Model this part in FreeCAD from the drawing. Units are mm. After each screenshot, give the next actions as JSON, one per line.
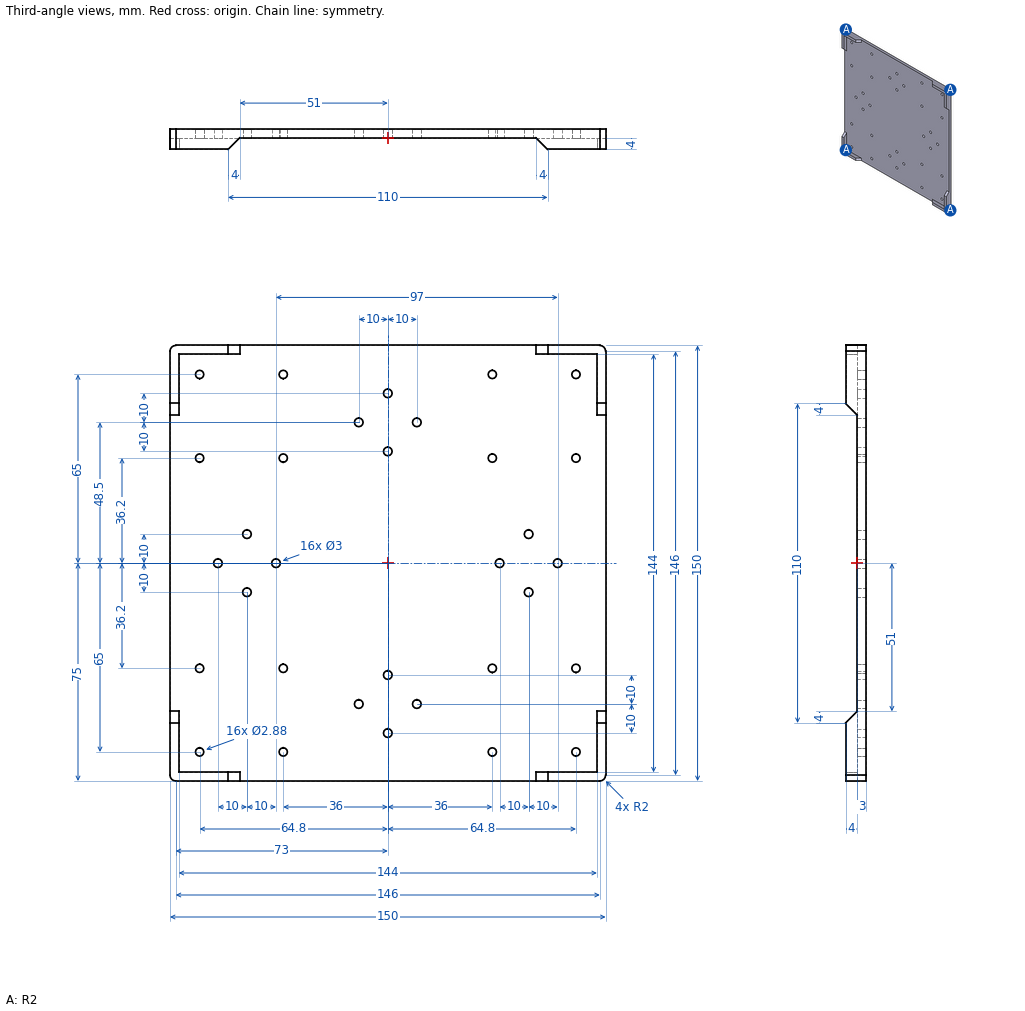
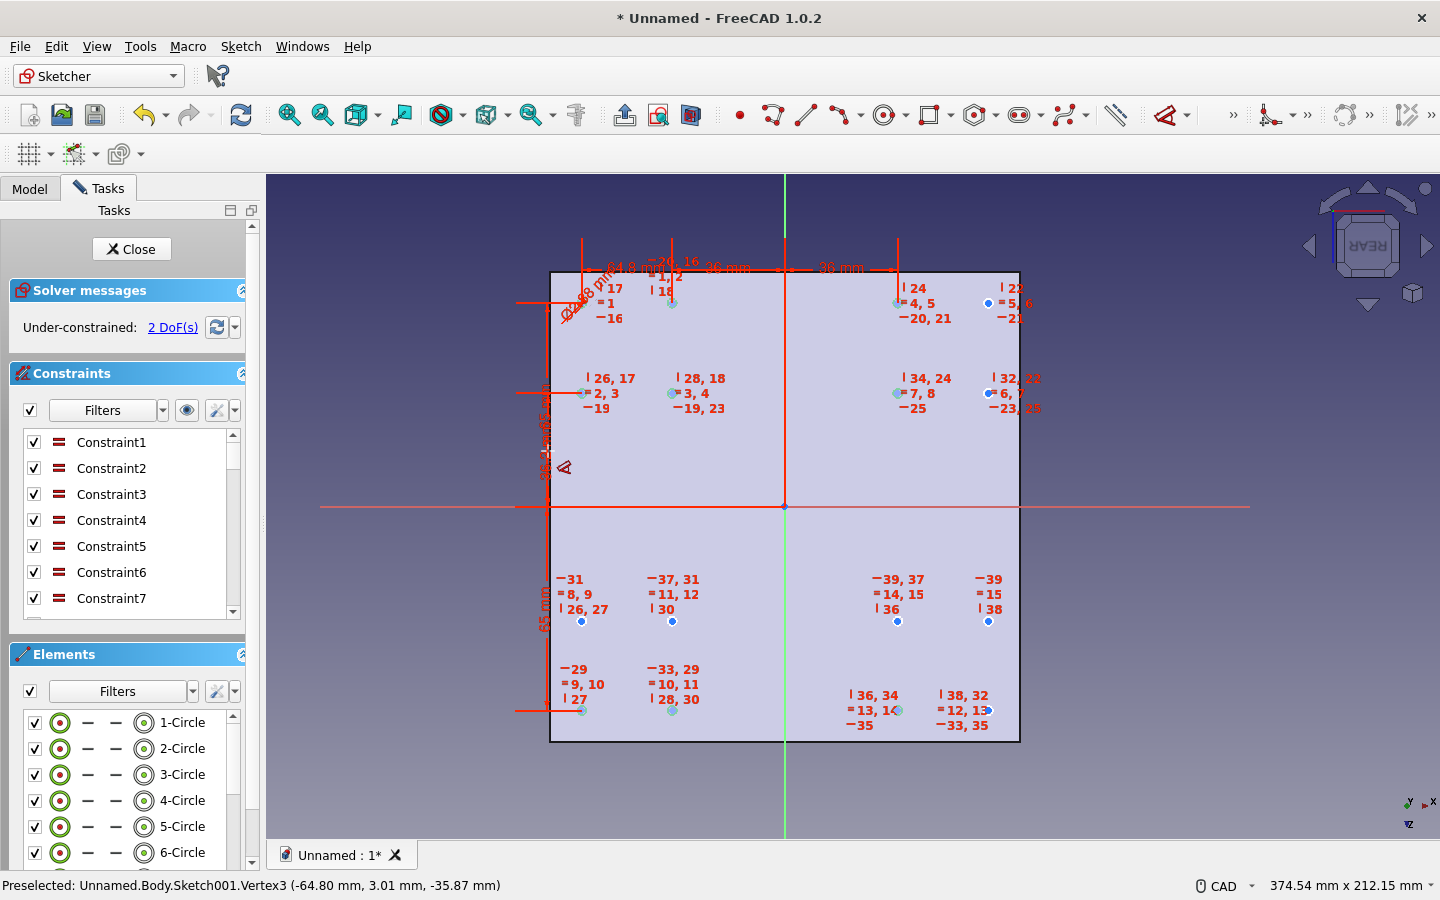
{"action": "left_click", "coordinate": [988, 303]}
{"action": "left_click", "coordinate": [933, 269]}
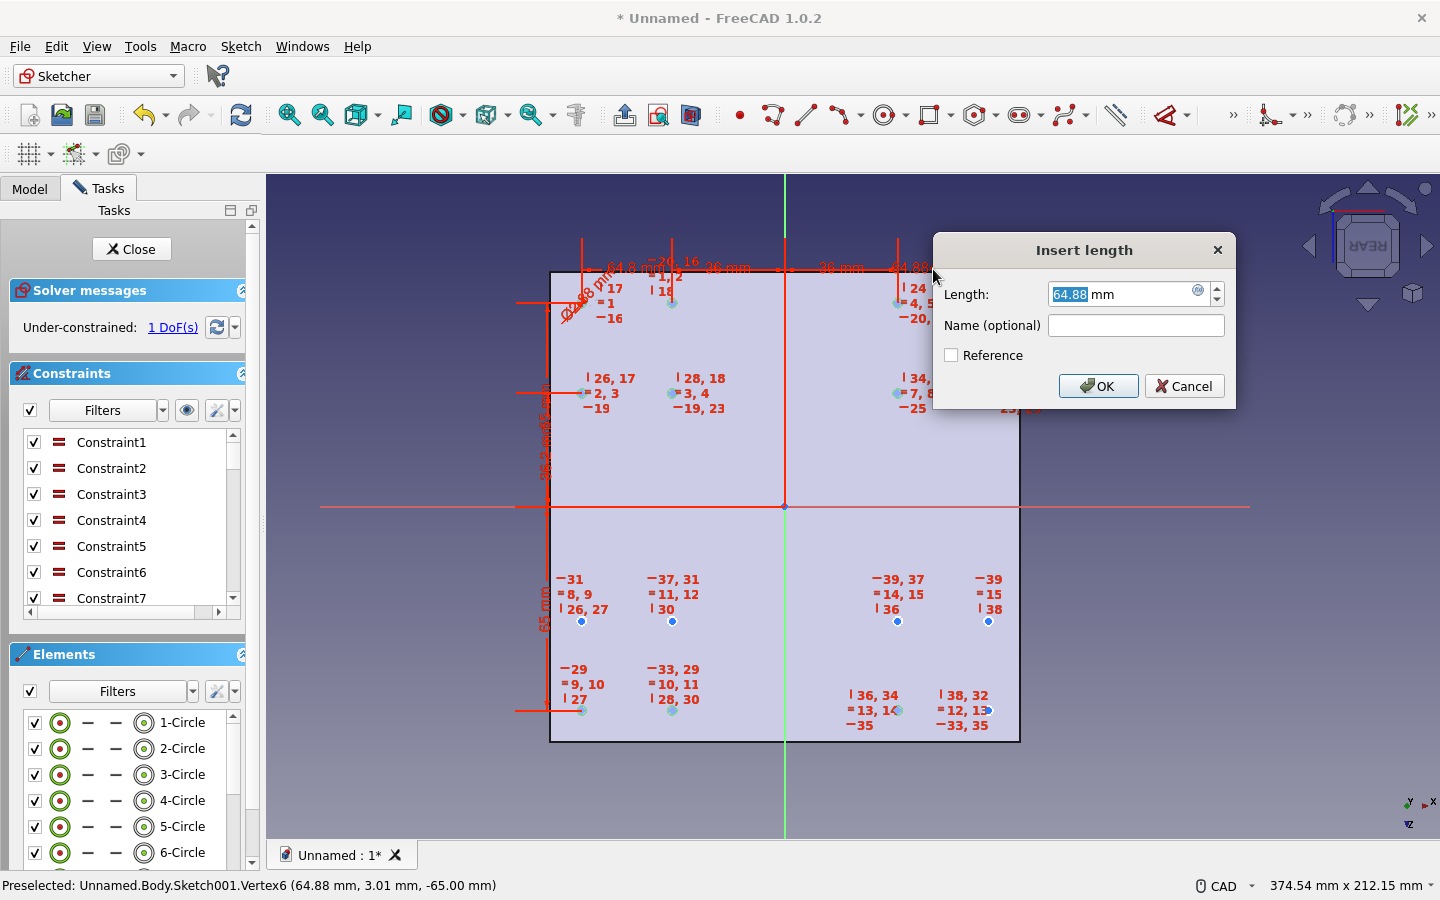
{"action": "type", "text": "64.8"}
{"action": "key", "text": "Return"}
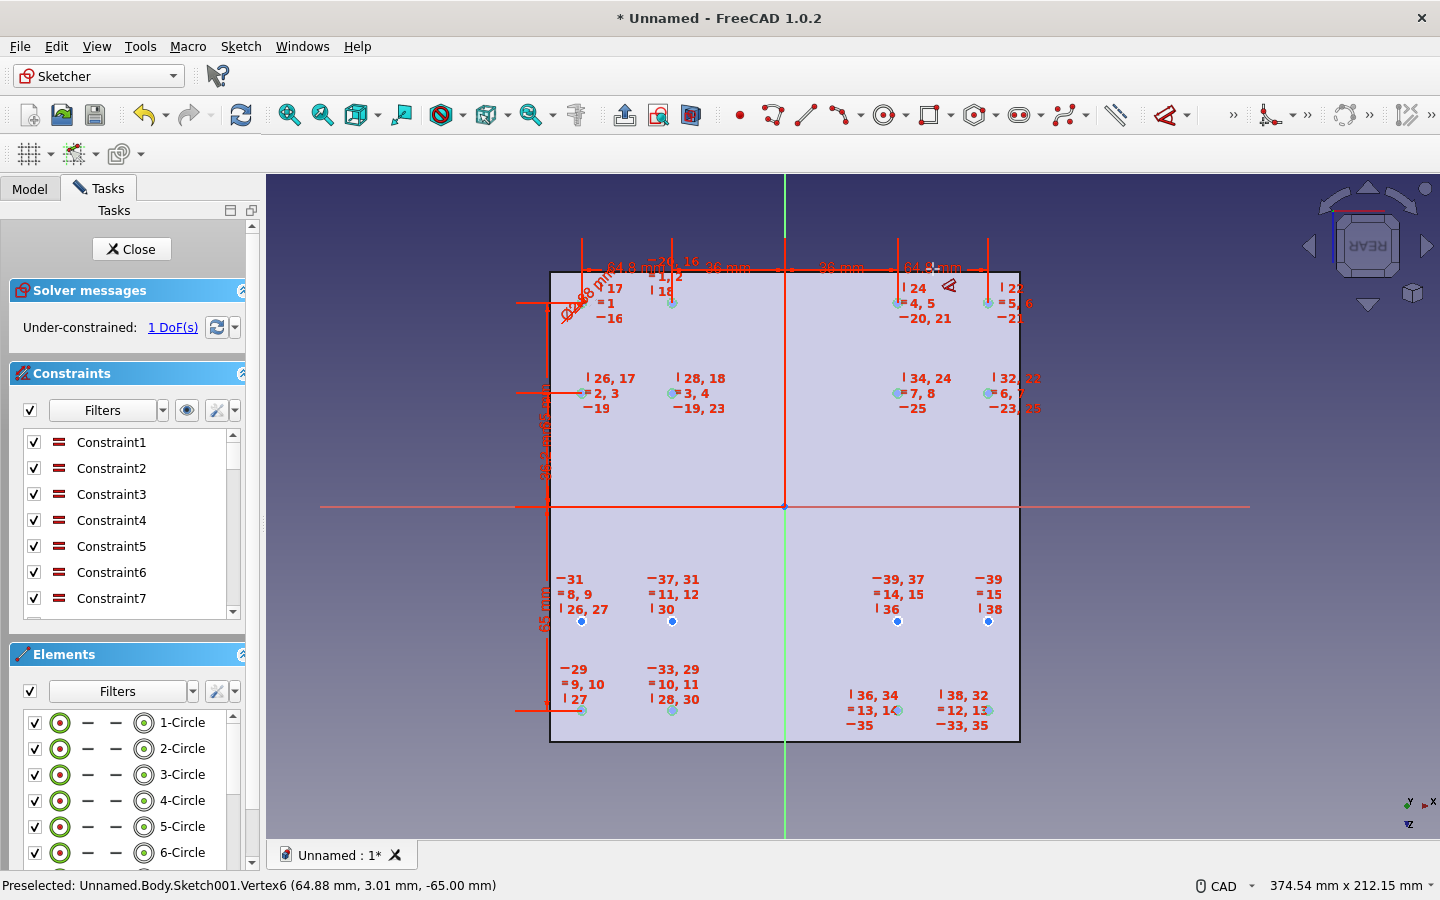
{"action": "left_click", "coordinate": [582, 621]}
{"action": "left_click", "coordinate": [548, 564]}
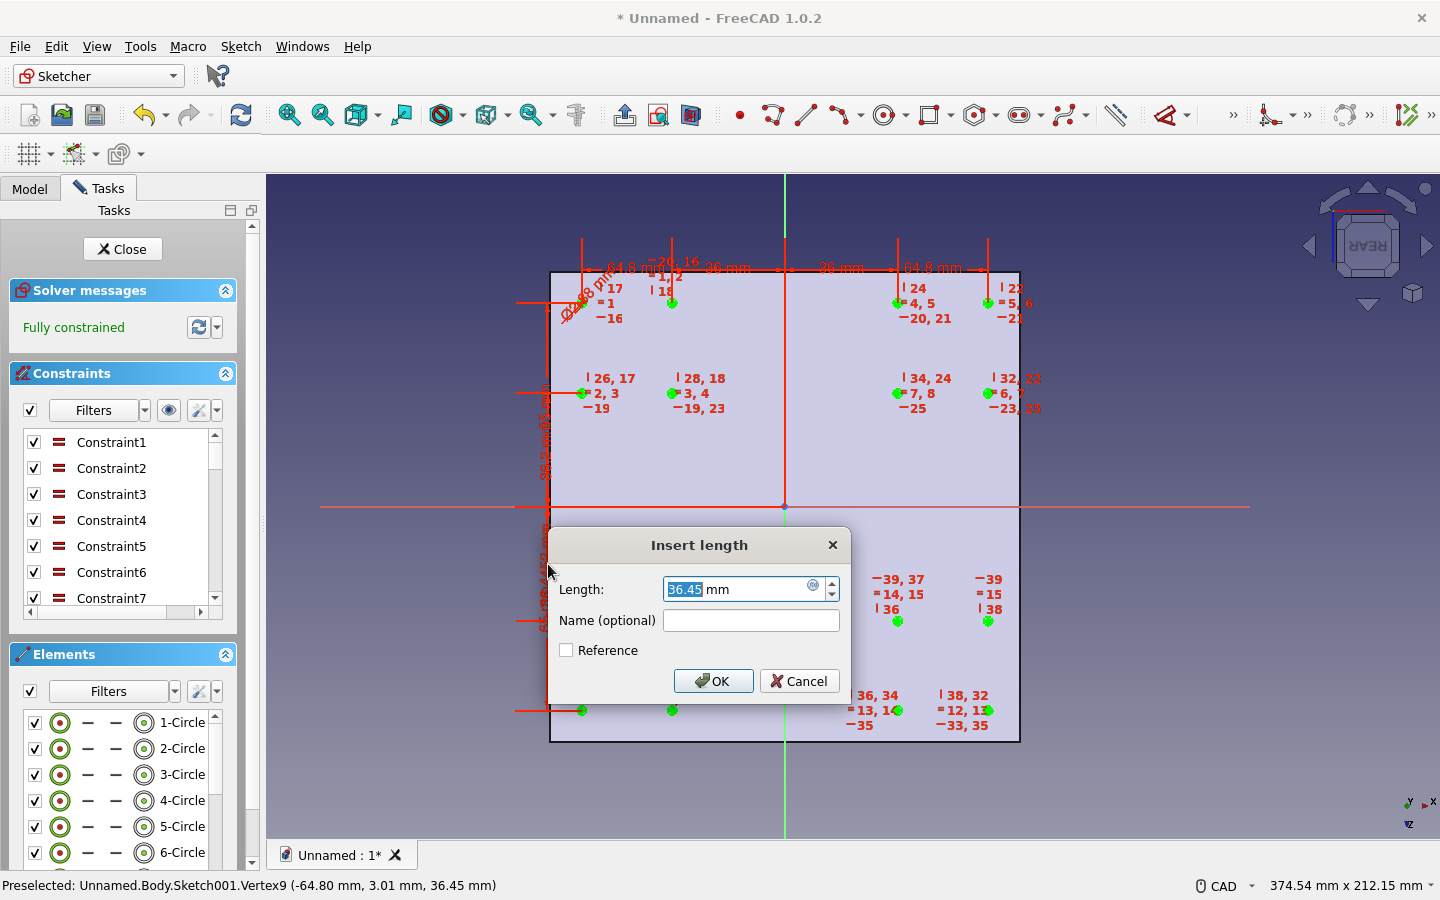
{"action": "type", "text": "36.2"}
{"action": "key", "text": "Return"}
{"action": "key", "text": "Escape"}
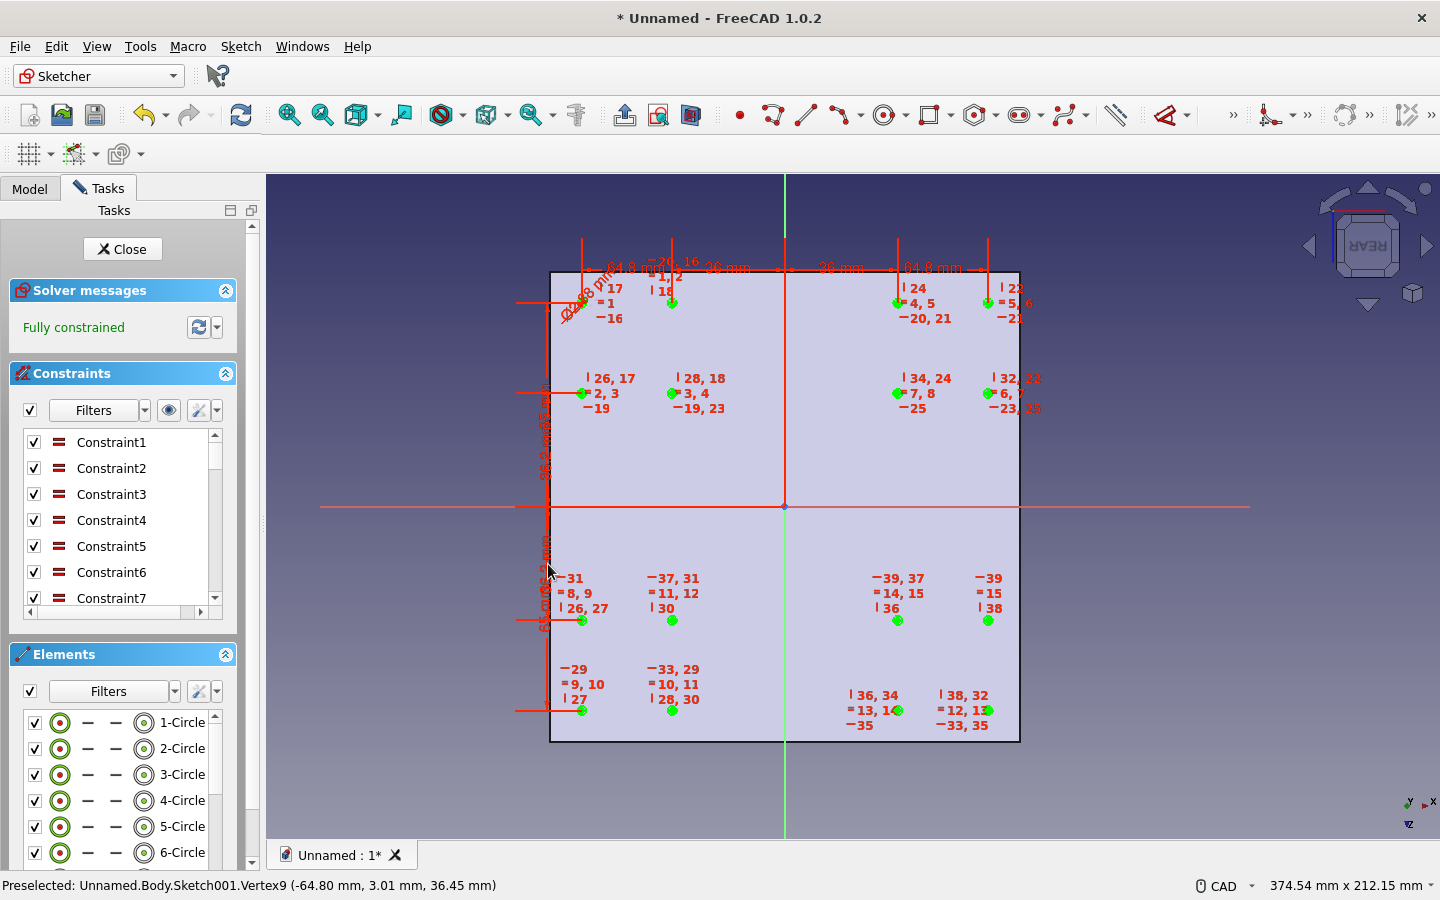
{"action": "left_click", "coordinate": [123, 249]}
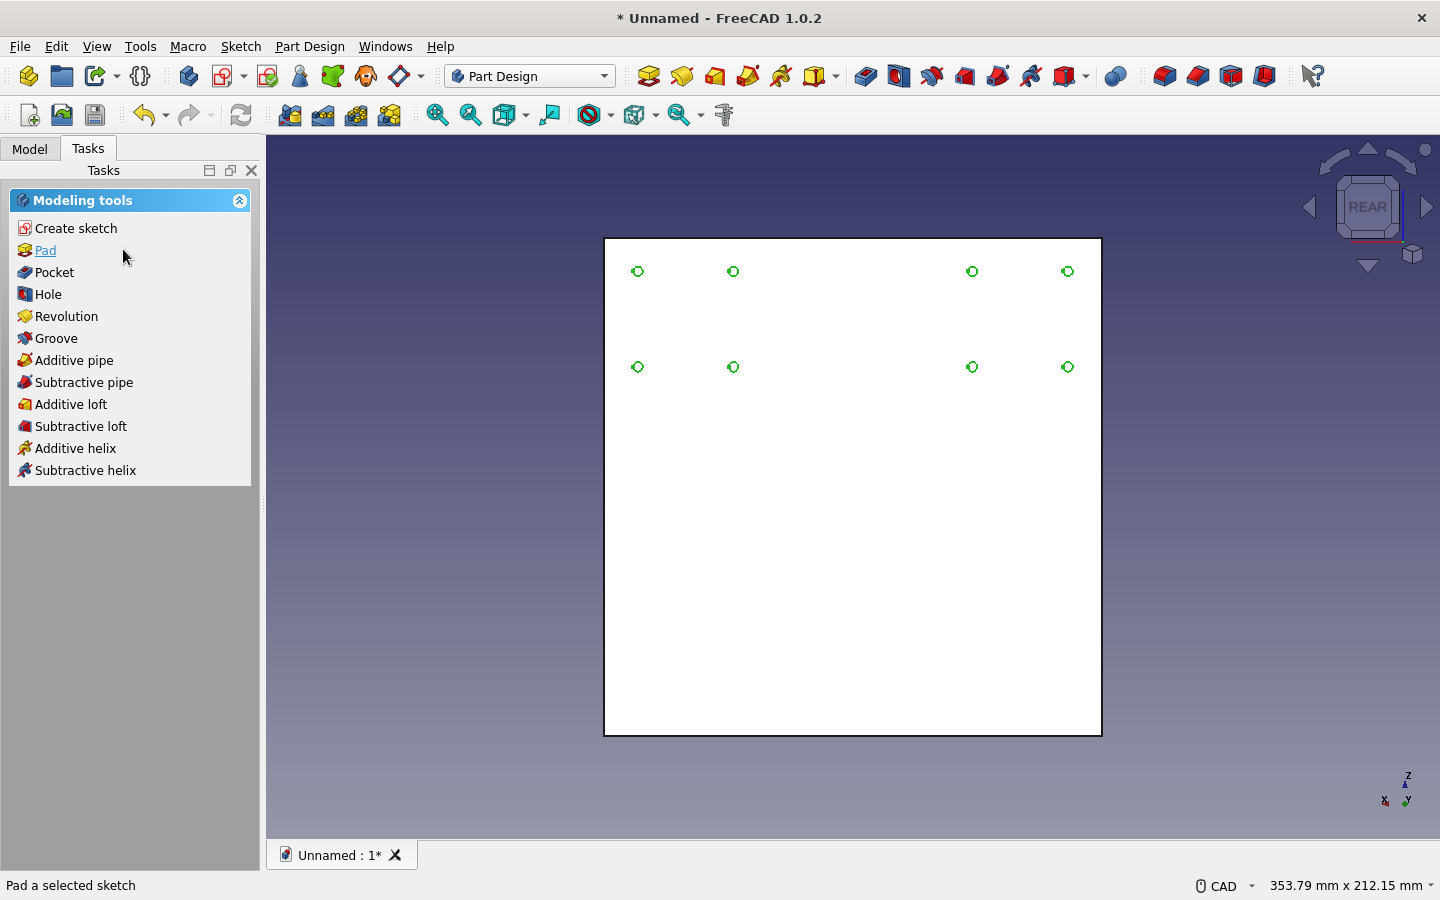
{"action": "left_click", "coordinate": [866, 76]}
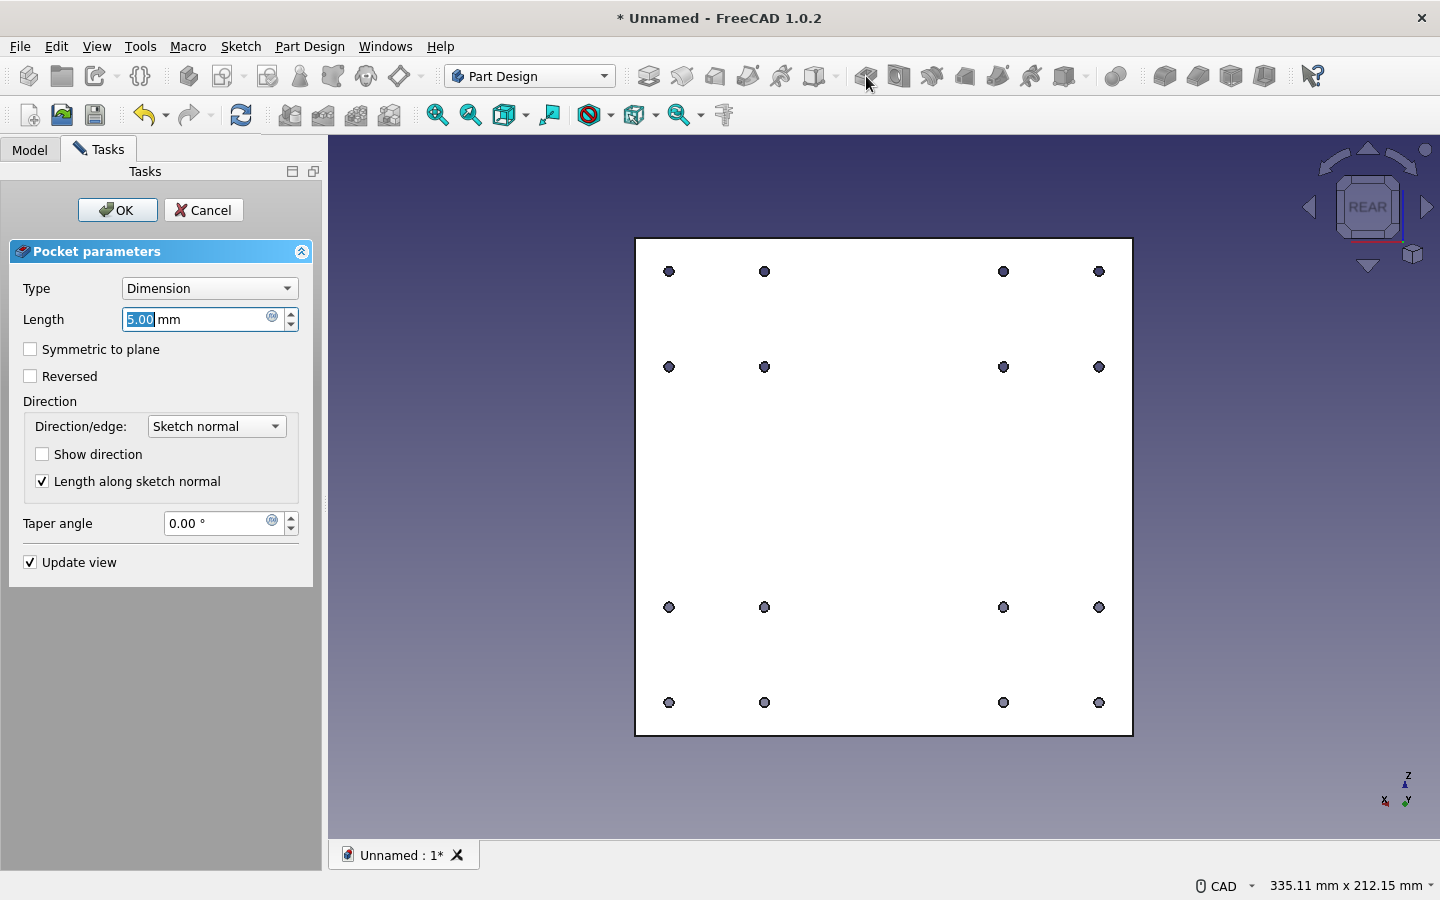
{"action": "left_click", "coordinate": [210, 288]}